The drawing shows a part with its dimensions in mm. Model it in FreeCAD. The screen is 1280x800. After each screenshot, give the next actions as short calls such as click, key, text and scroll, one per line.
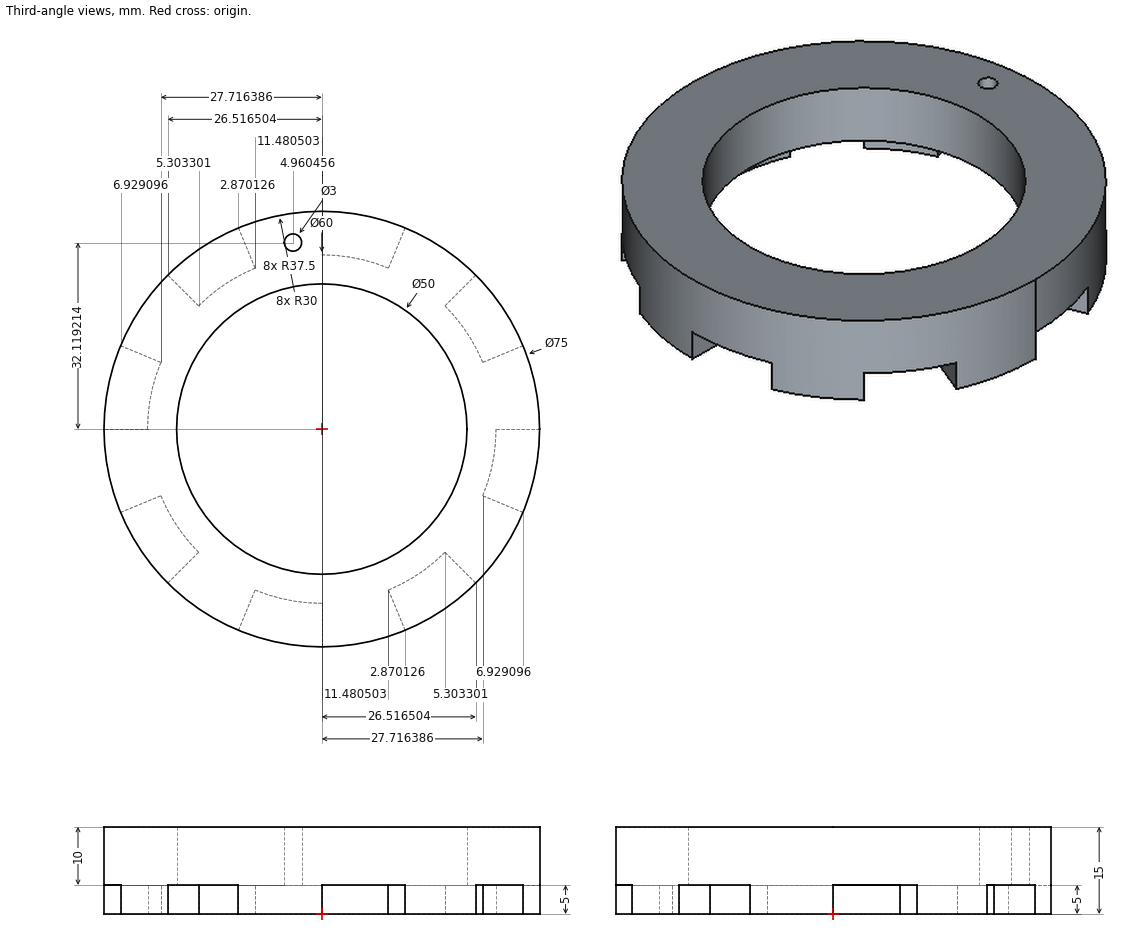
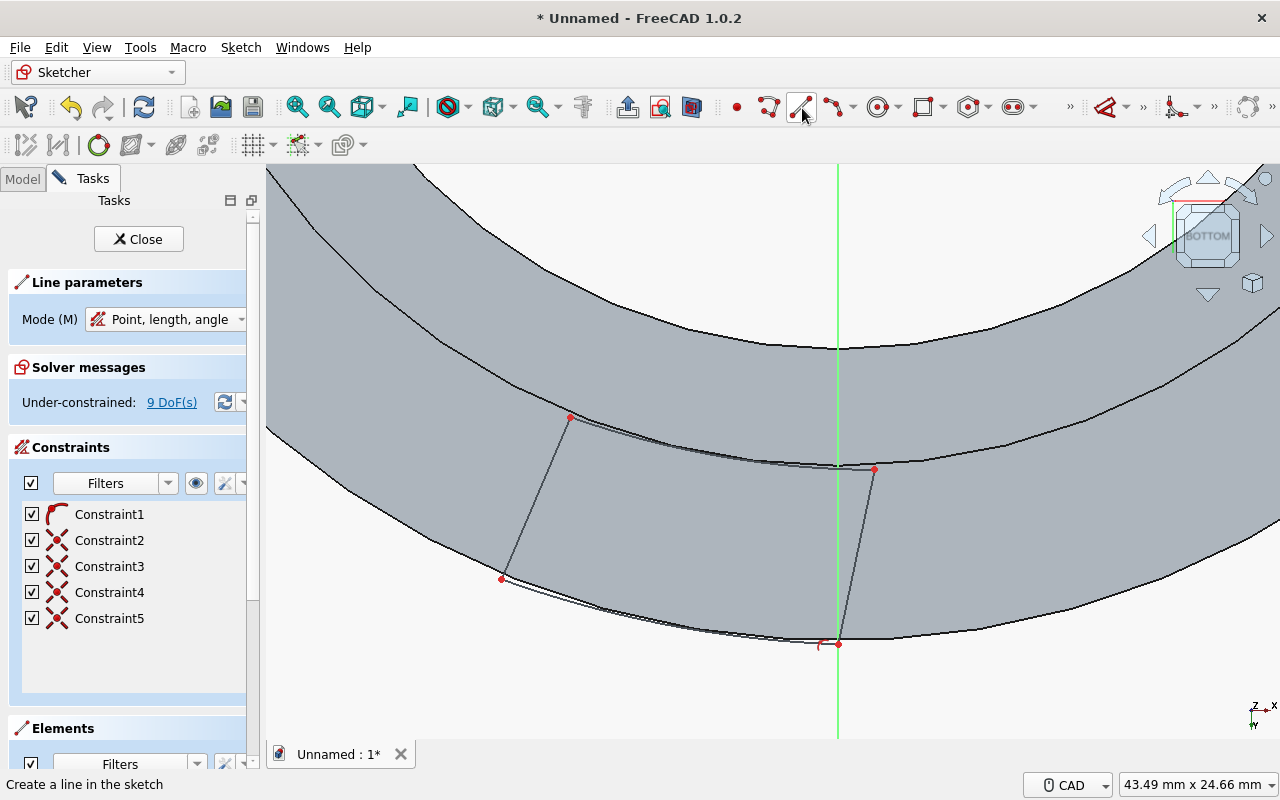
scroll(671, 625, down, 8)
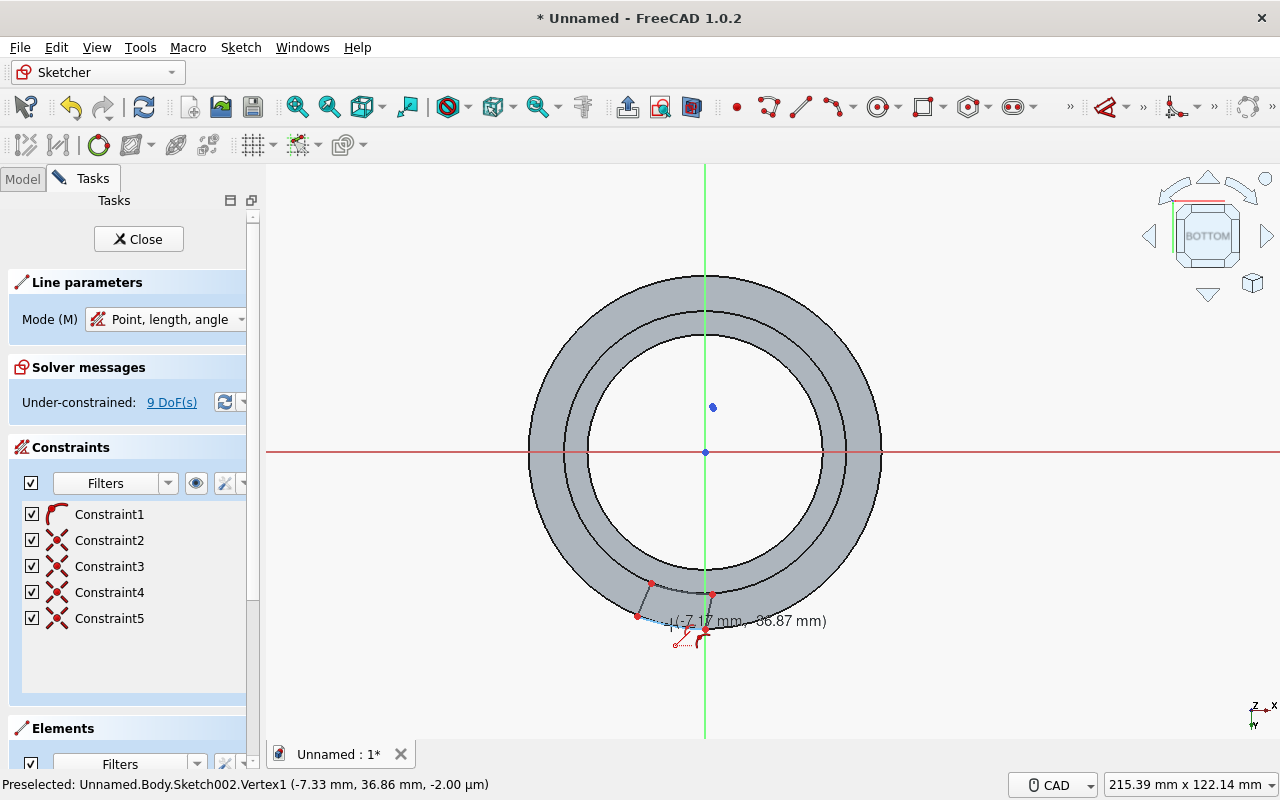
click(580, 577)
click(605, 552)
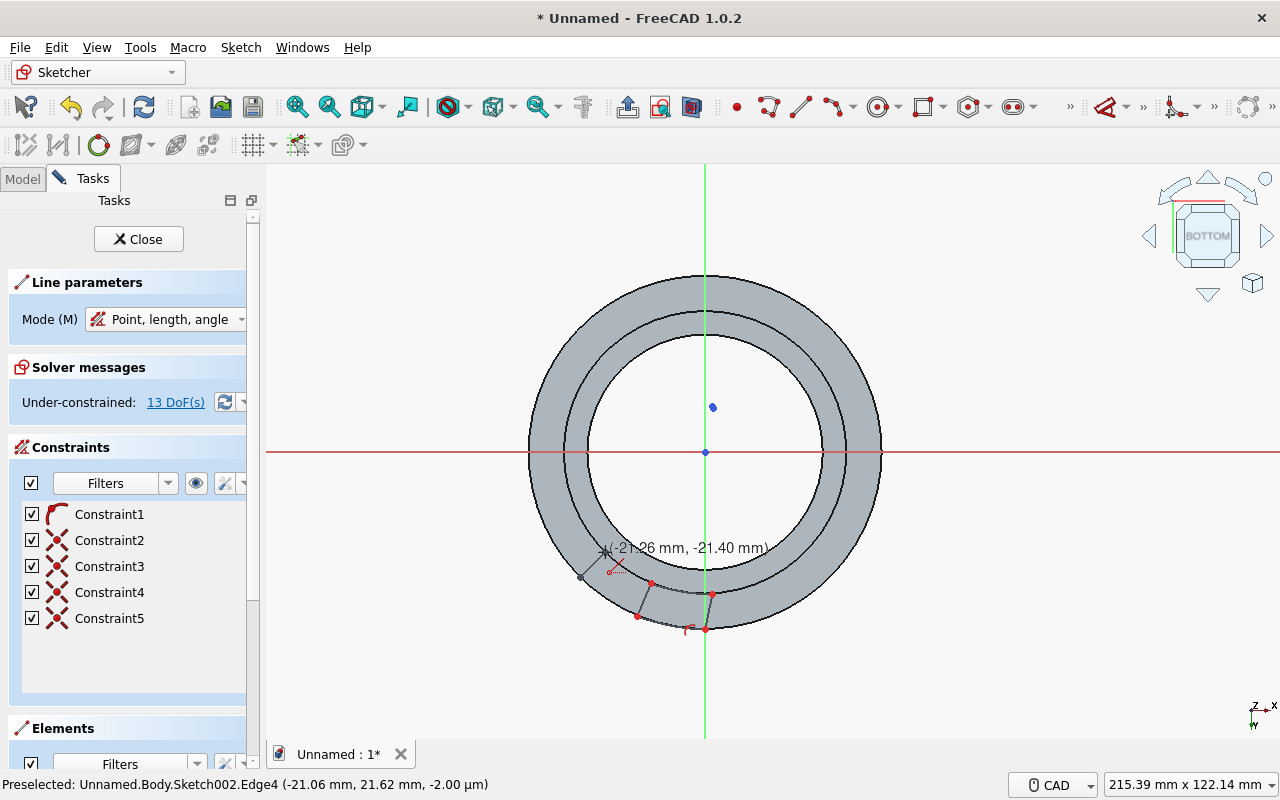
click(575, 506)
click(542, 520)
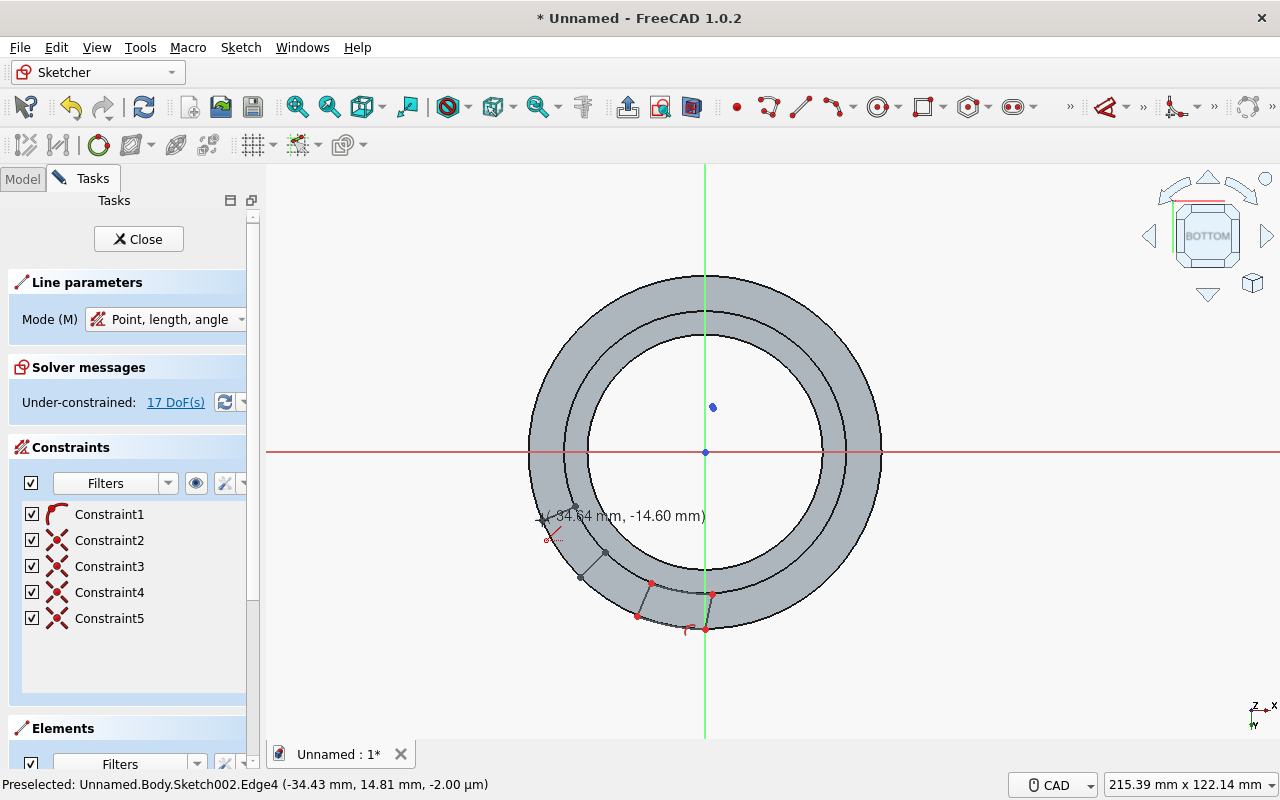
click(834, 108)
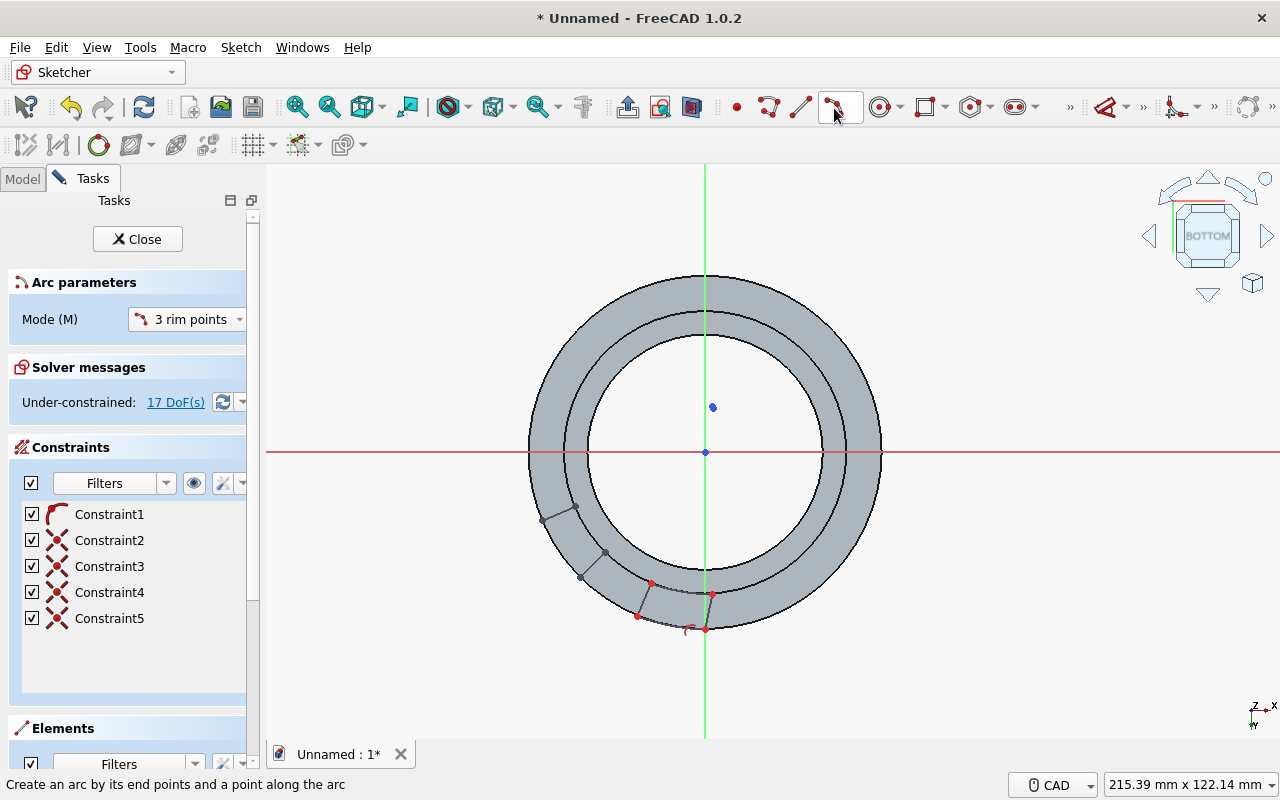
click(605, 553)
click(575, 507)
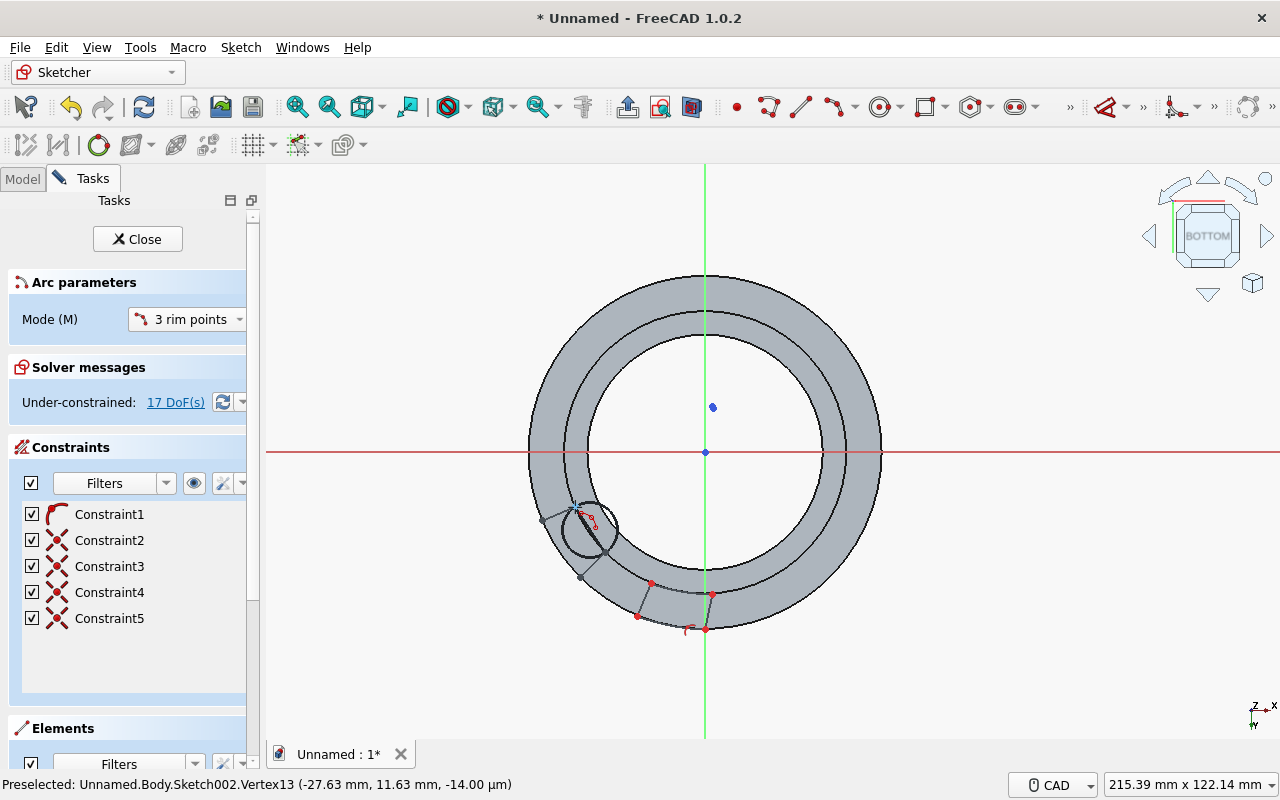
scroll(588, 531, up, 9)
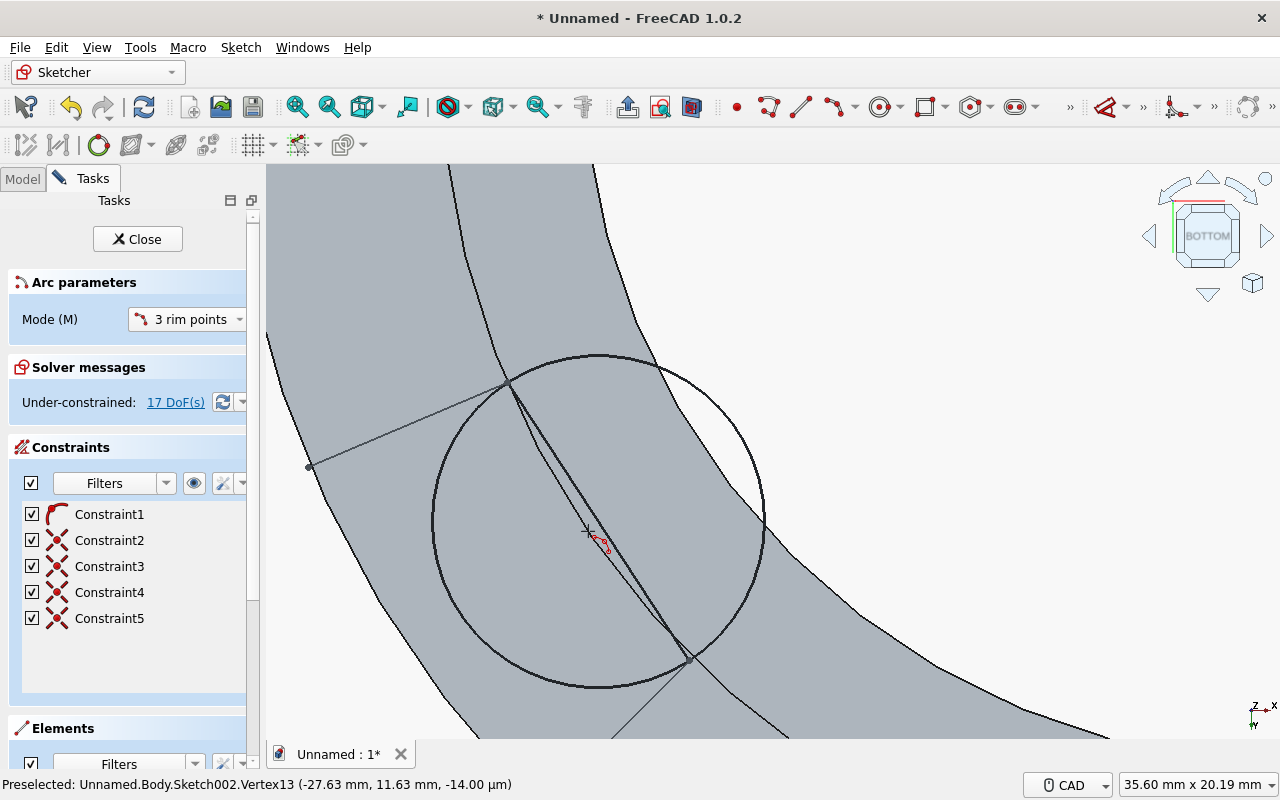
click(584, 526)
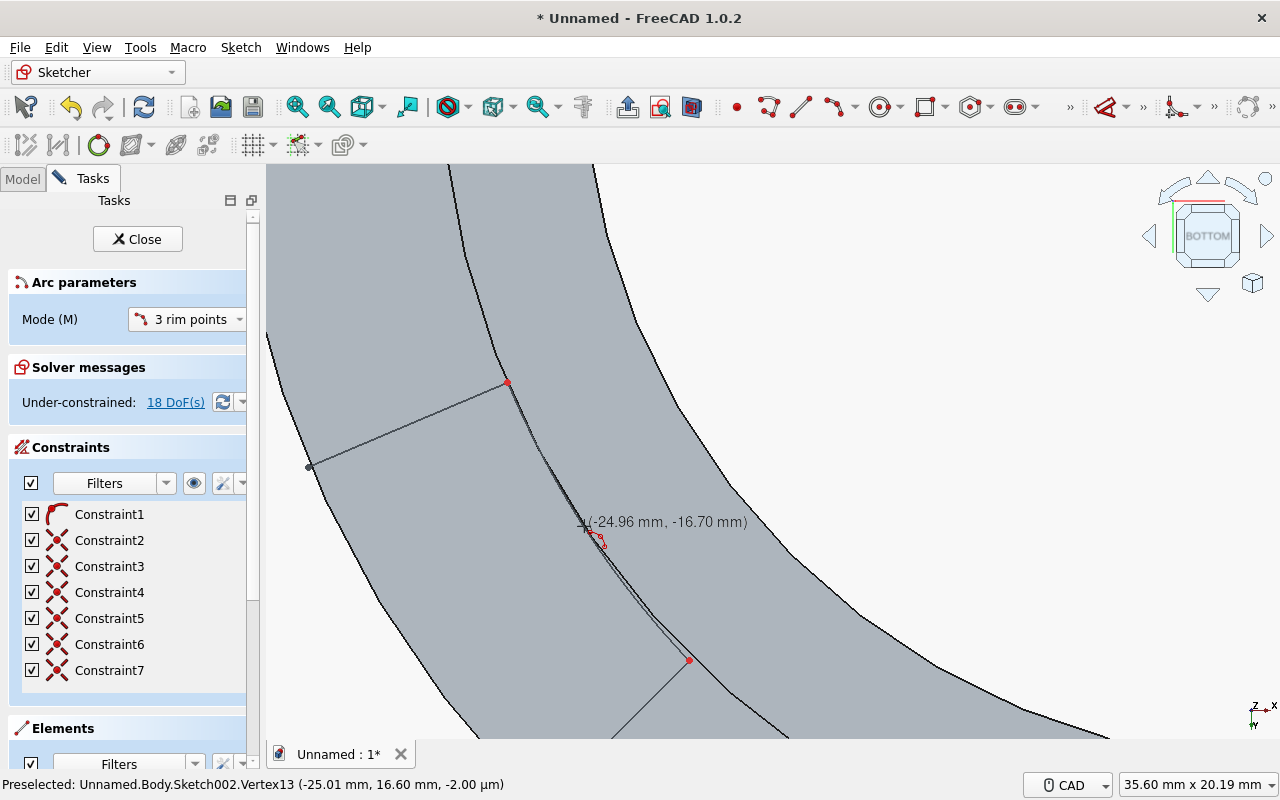
scroll(588, 531, down, 9)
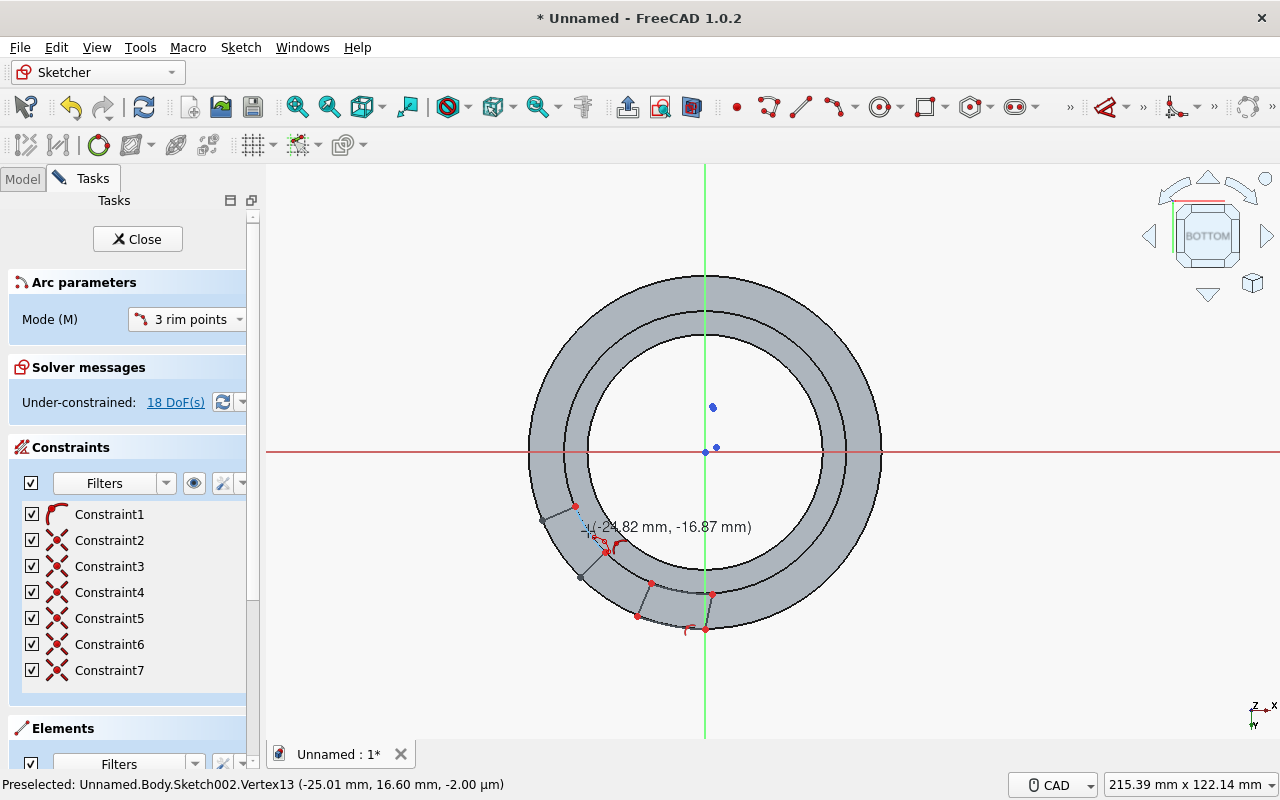
click(542, 521)
click(580, 578)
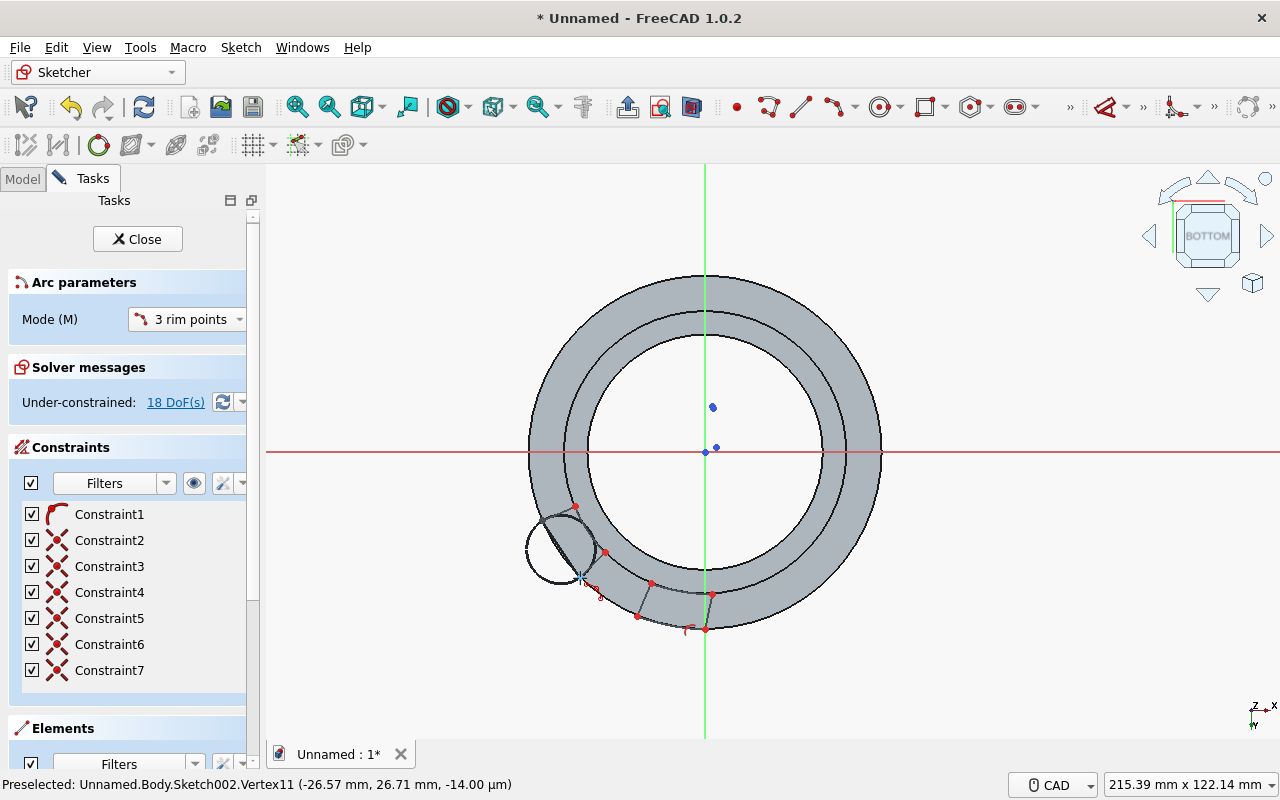
scroll(558, 550, up, 8)